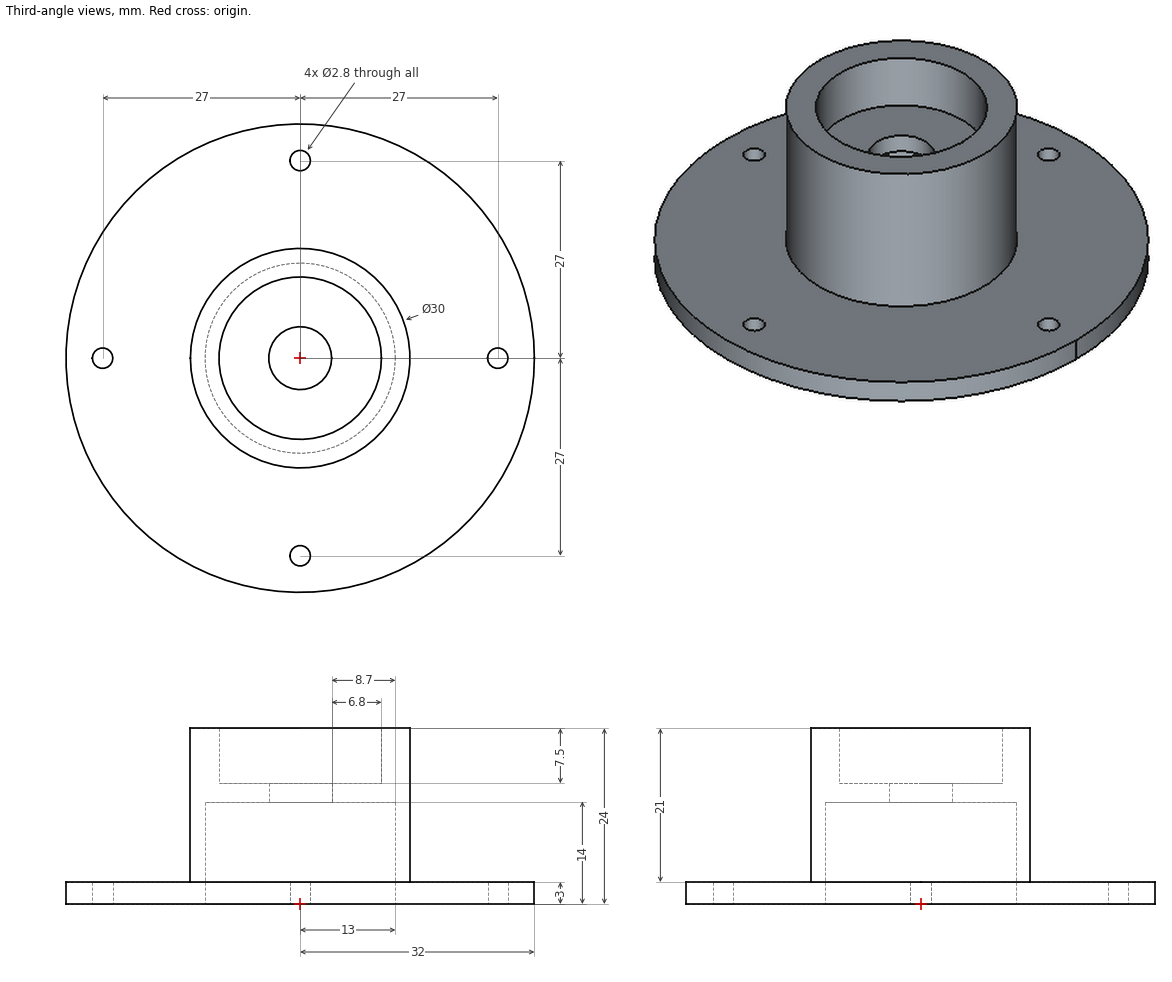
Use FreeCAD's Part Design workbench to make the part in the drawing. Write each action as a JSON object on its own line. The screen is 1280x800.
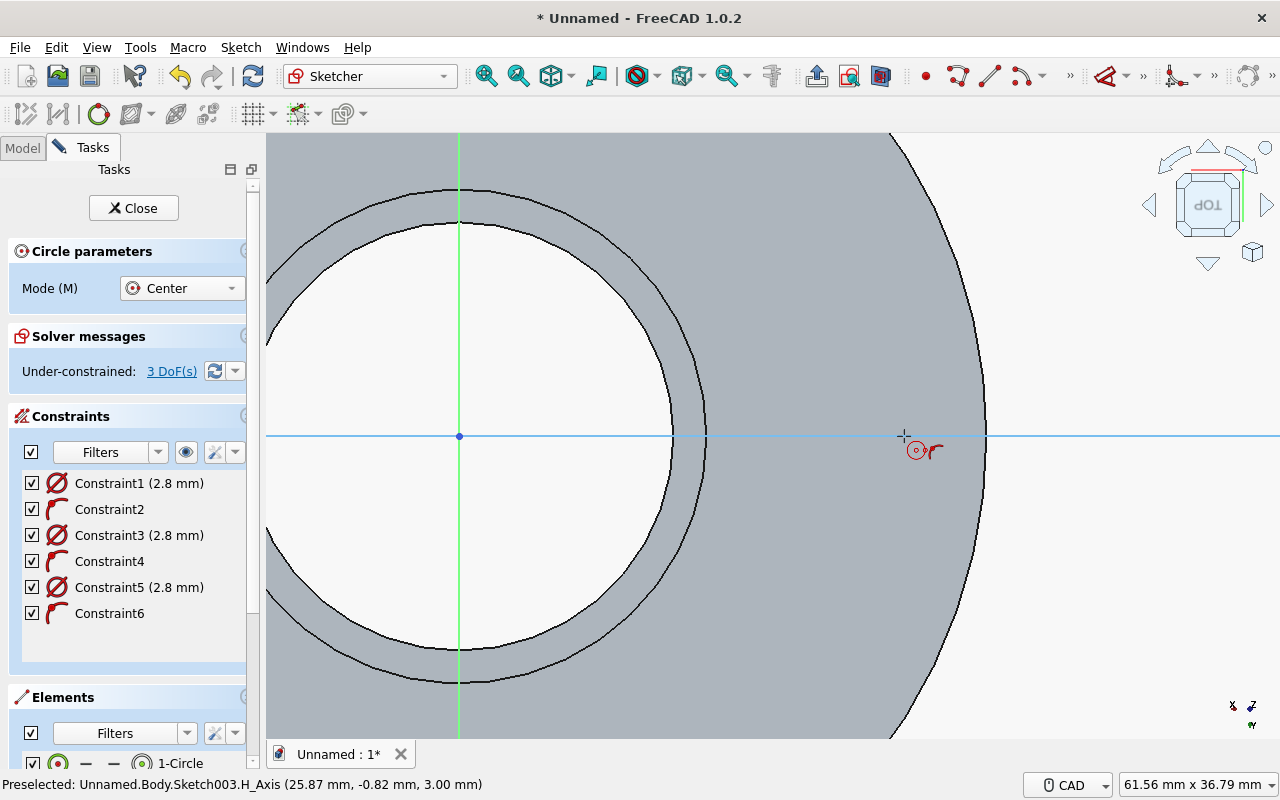
{"action": "left_click", "coordinate": [904, 436]}
{"action": "mouse_move", "coordinate": [920, 420]}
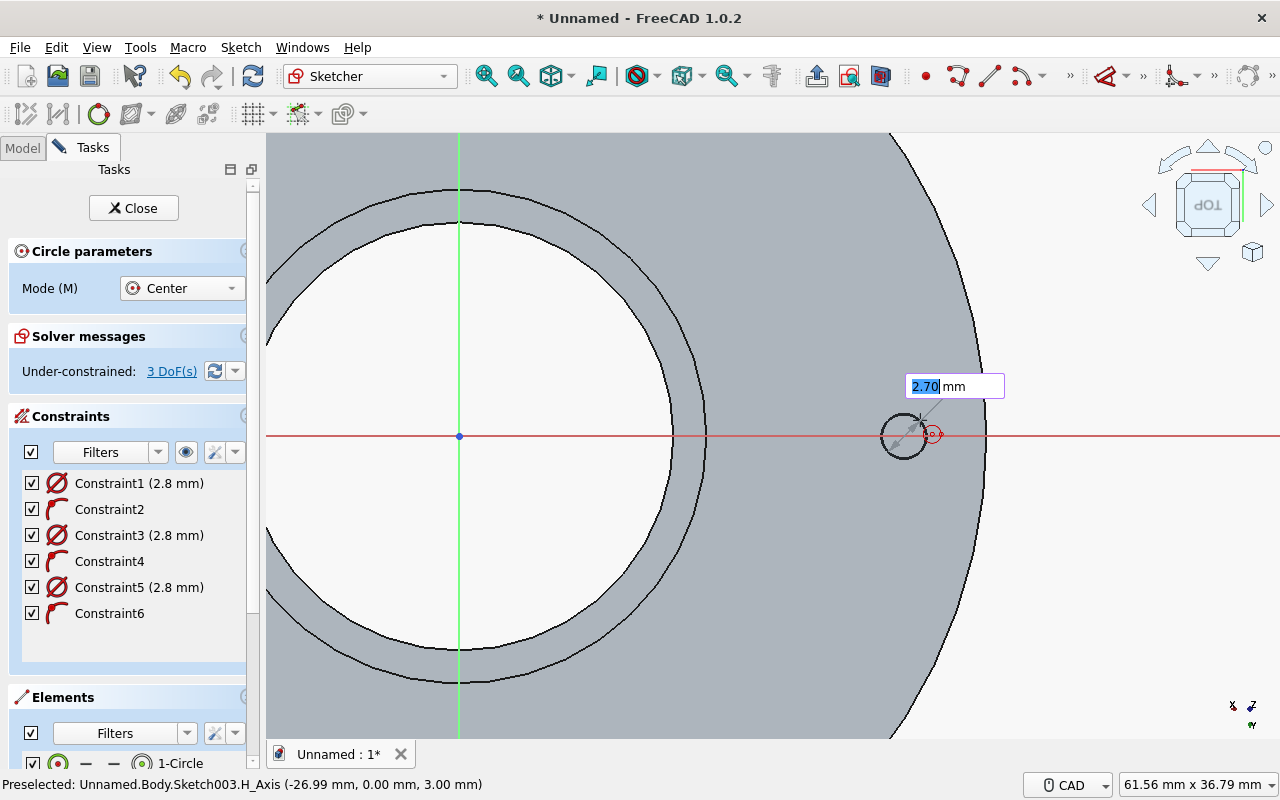
{"action": "type", "text": "2.8"}
{"action": "key", "text": "Return"}
{"action": "key", "text": "Escape"}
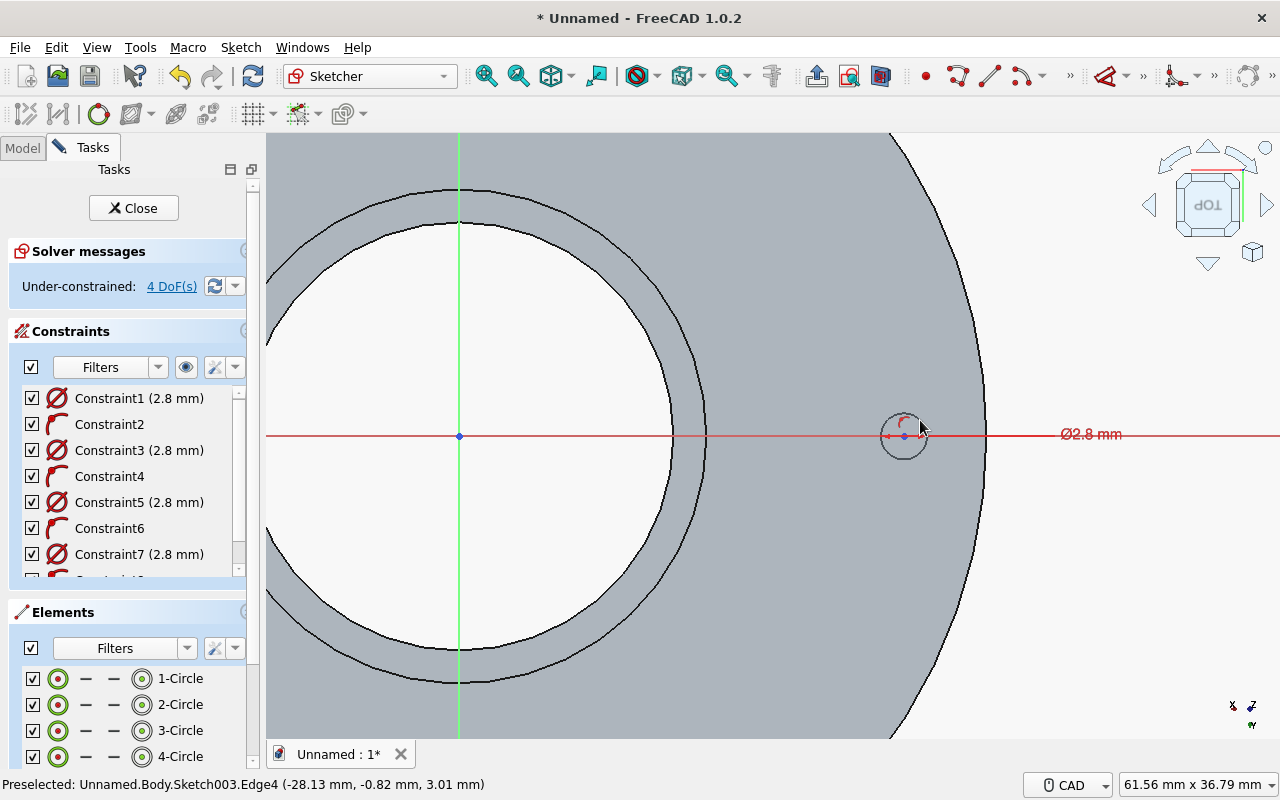
{"action": "left_click", "coordinate": [1106, 76]}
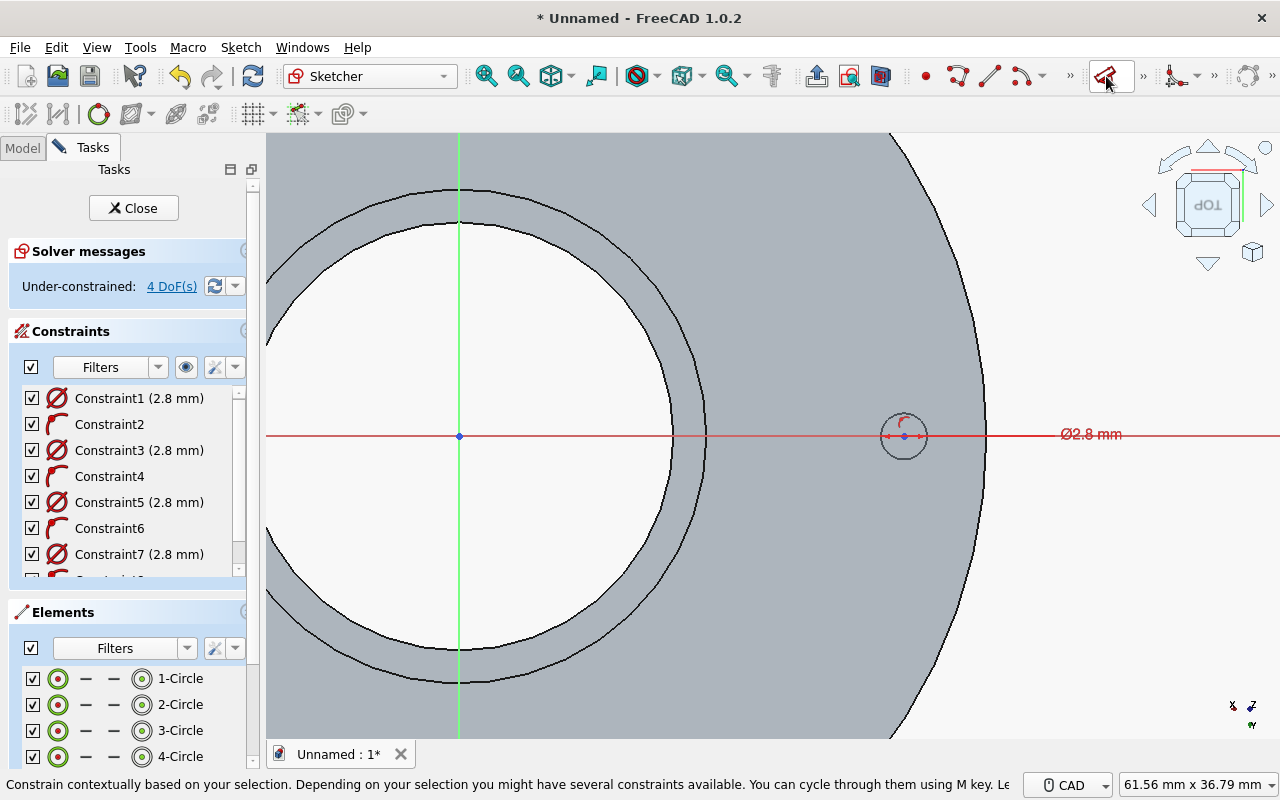
{"action": "scroll", "coordinate": [905, 436], "scroll_direction": "down", "scroll_amount": 4}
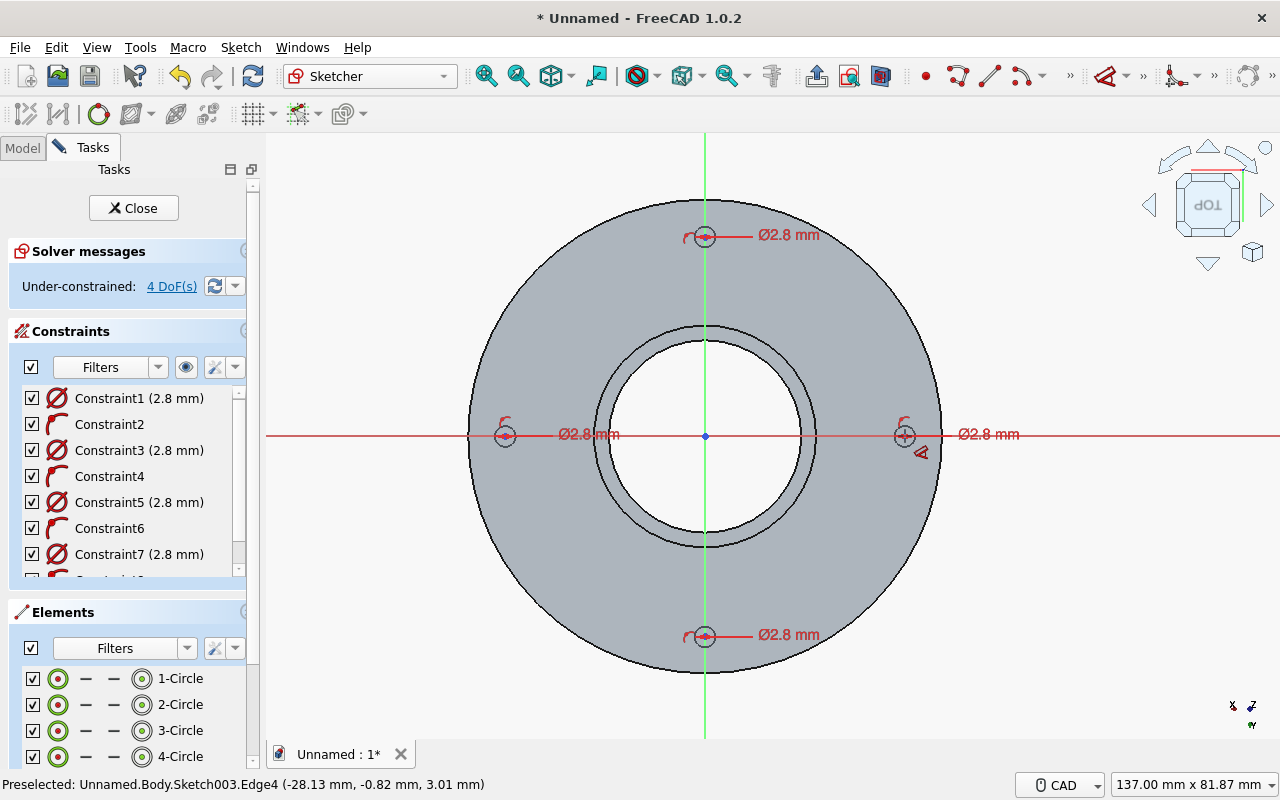
{"action": "left_click", "coordinate": [705, 637]}
{"action": "left_click", "coordinate": [739, 537]}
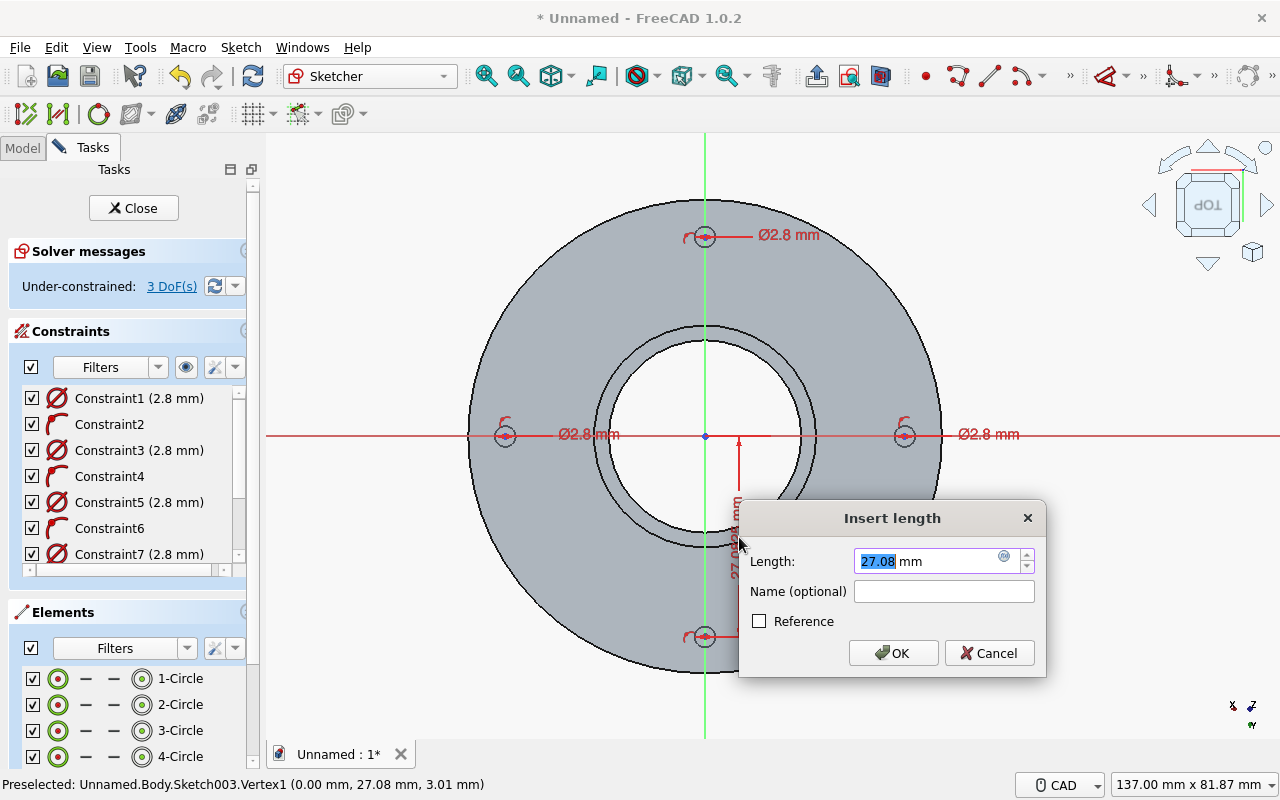
{"action": "type", "text": "27"}
{"action": "key", "text": "Return"}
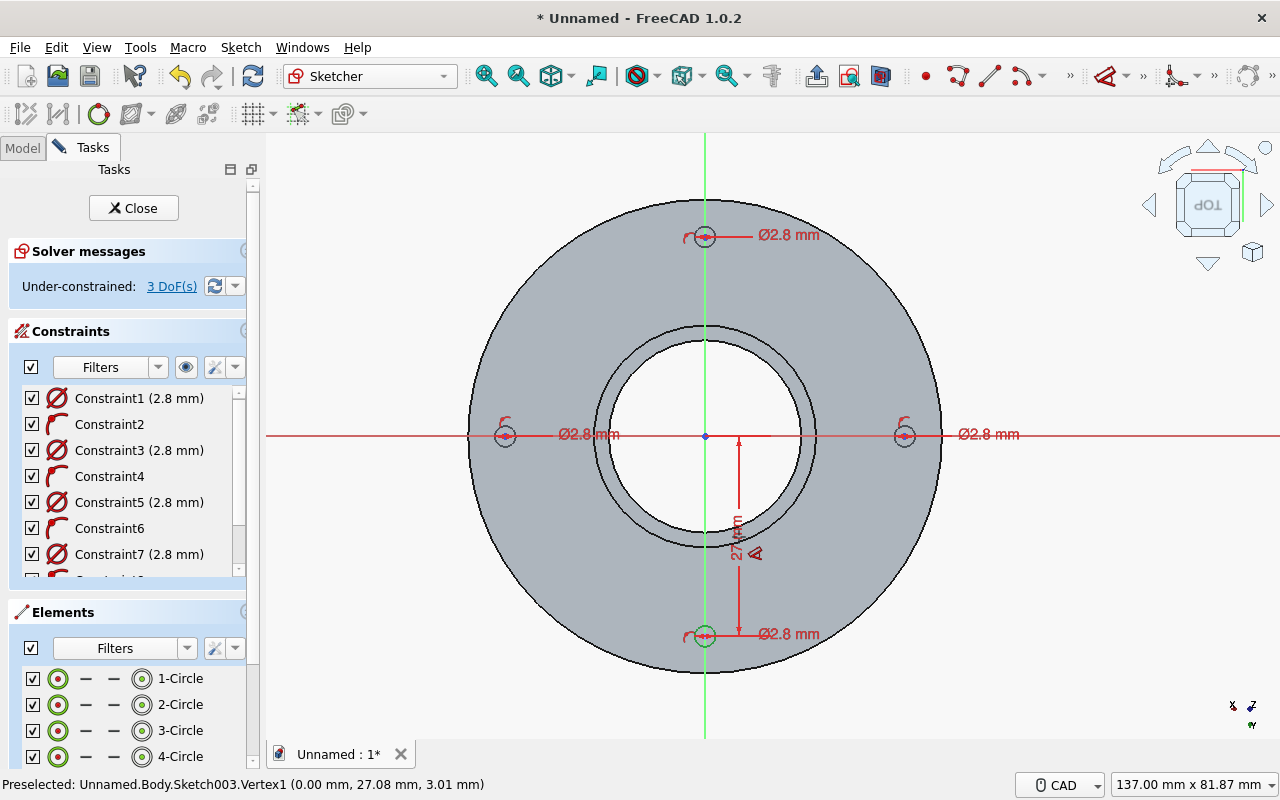
{"action": "left_click", "coordinate": [705, 237]}
{"action": "left_click", "coordinate": [739, 337]}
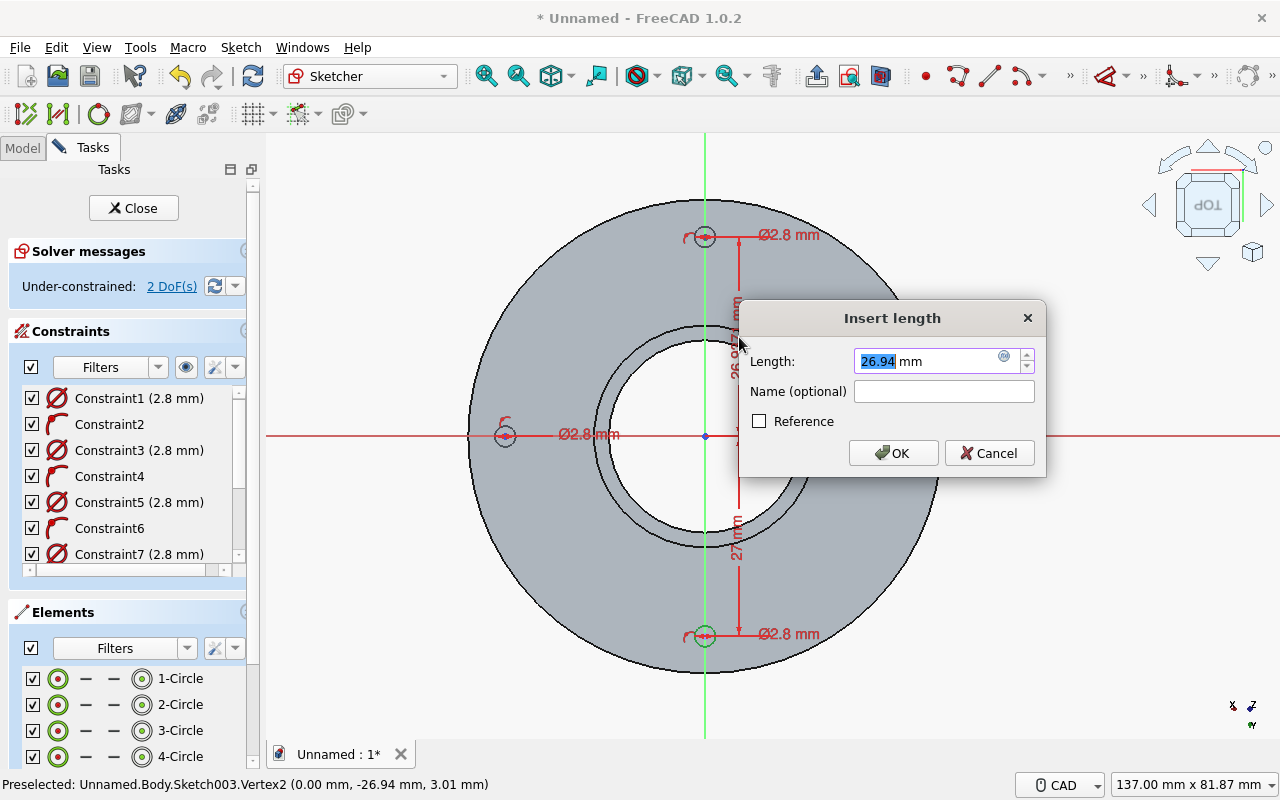
{"action": "type", "text": "27"}
{"action": "key", "text": "Return"}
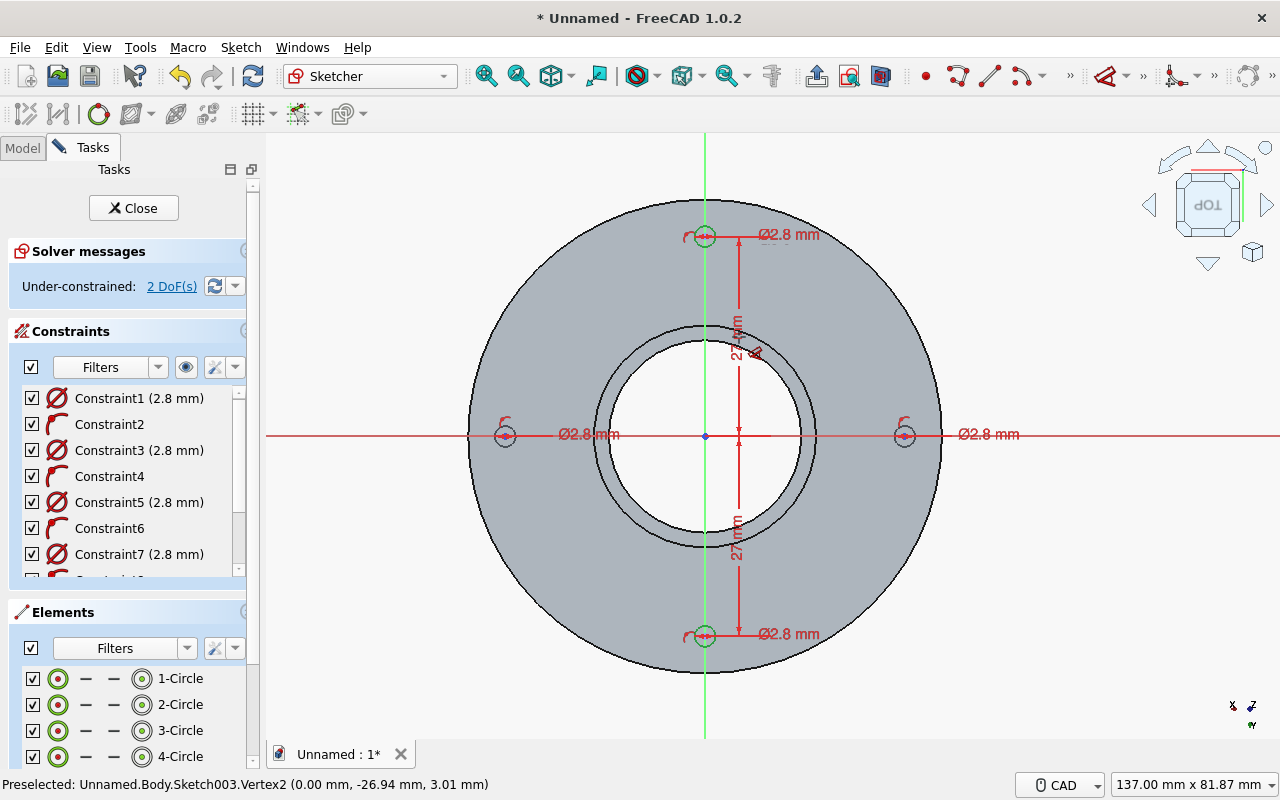
{"action": "left_click", "coordinate": [505, 436]}
{"action": "left_click", "coordinate": [605, 470]}